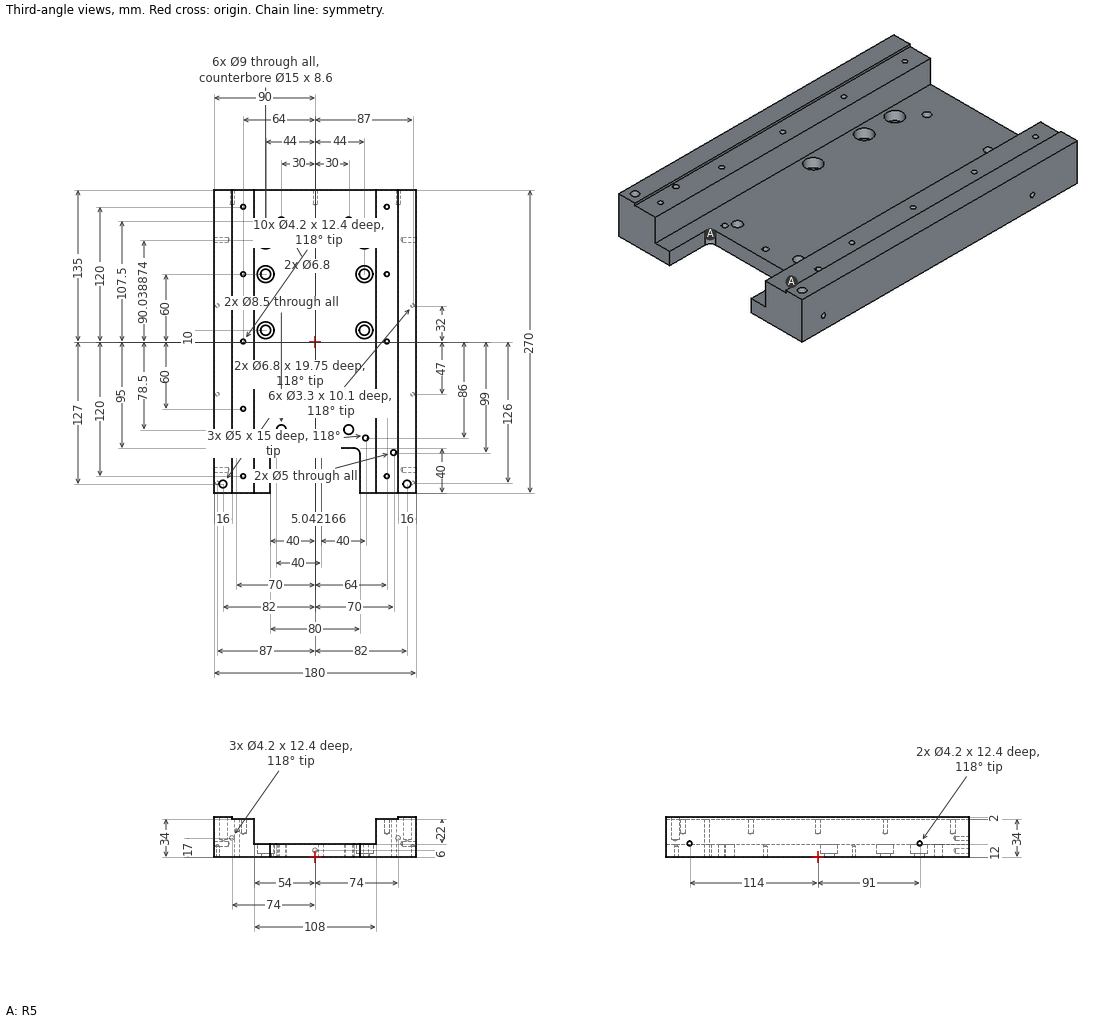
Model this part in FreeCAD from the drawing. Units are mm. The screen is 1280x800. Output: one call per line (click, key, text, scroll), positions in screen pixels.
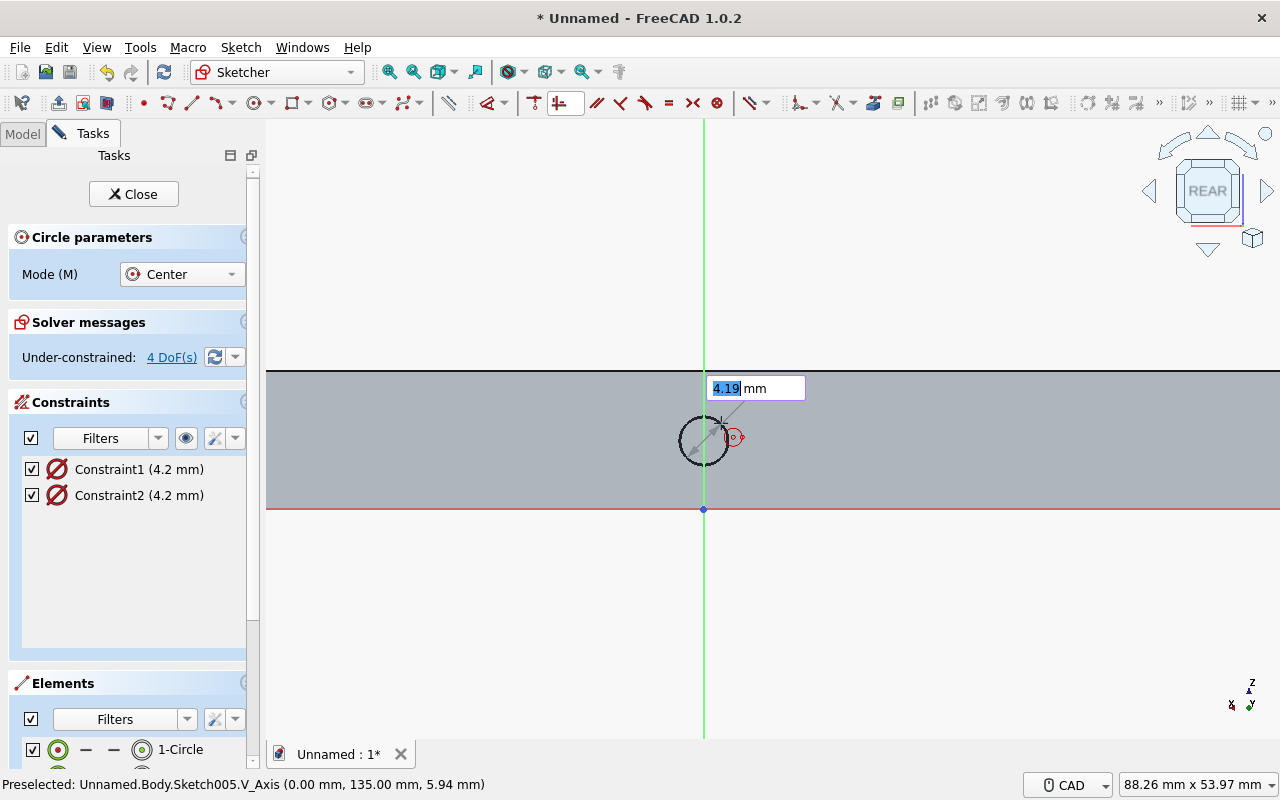
text(4.2)
key(Return)
key(Escape)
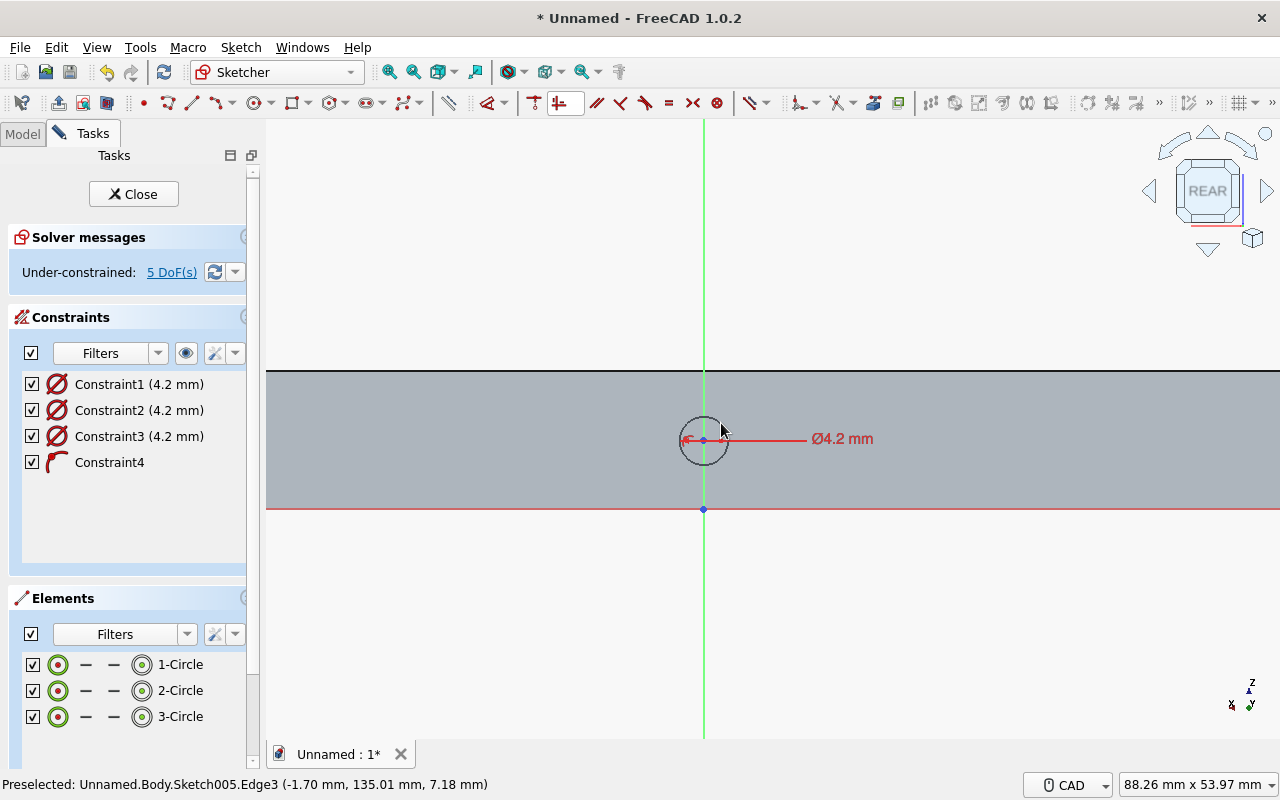
scroll(705, 442, down, 6)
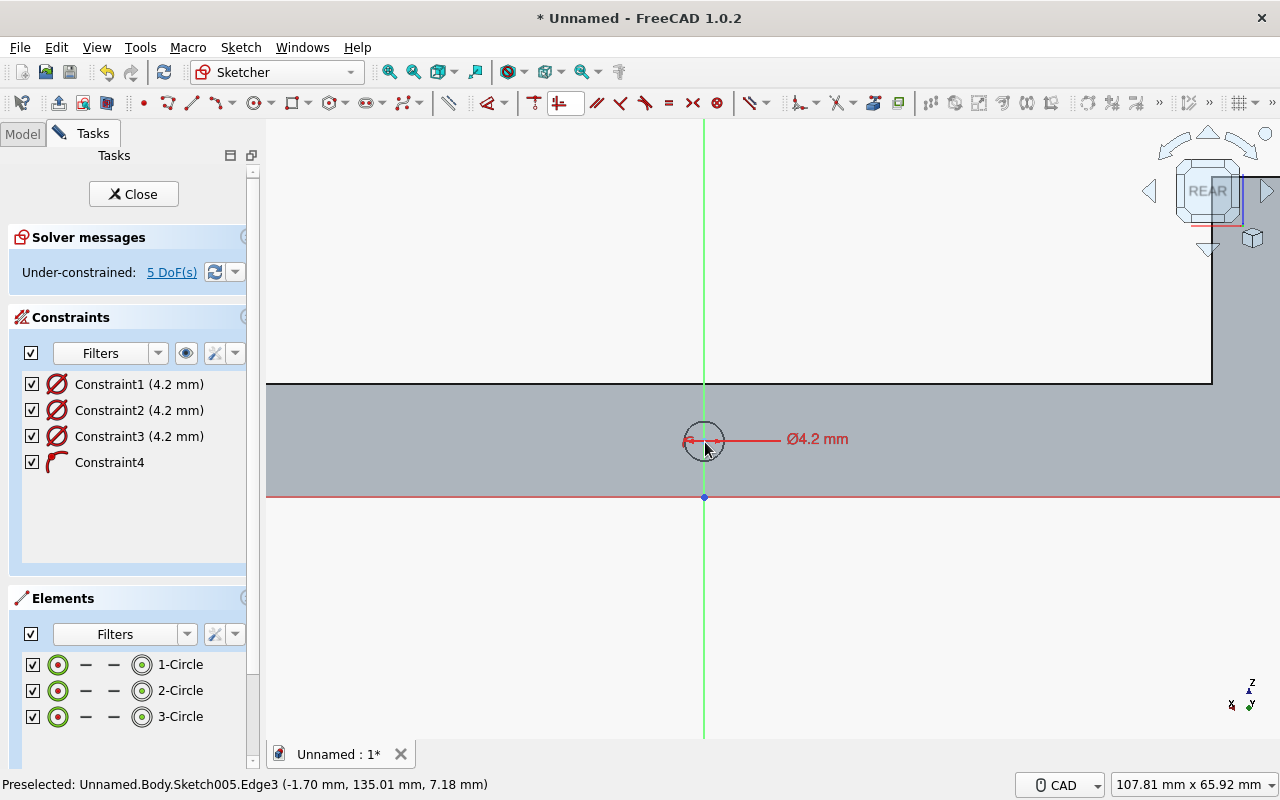
click(961, 404)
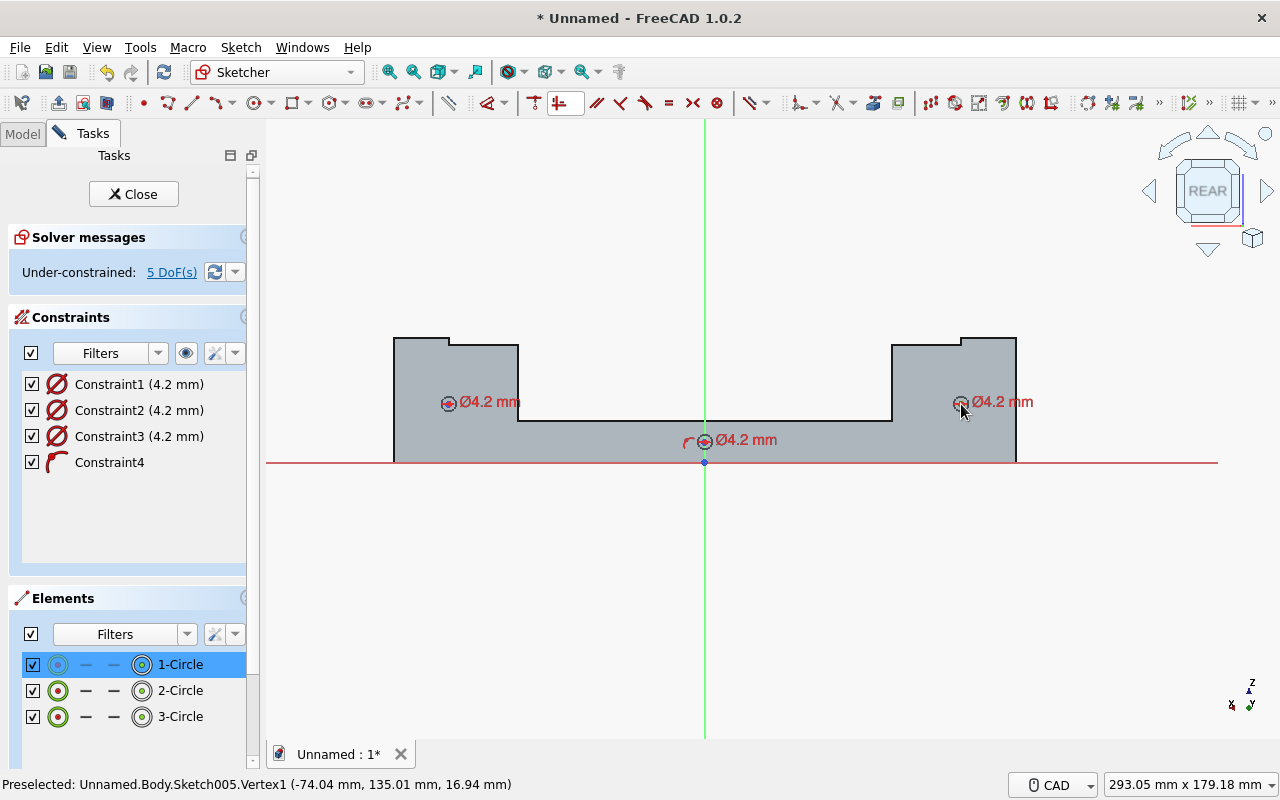
click(449, 404)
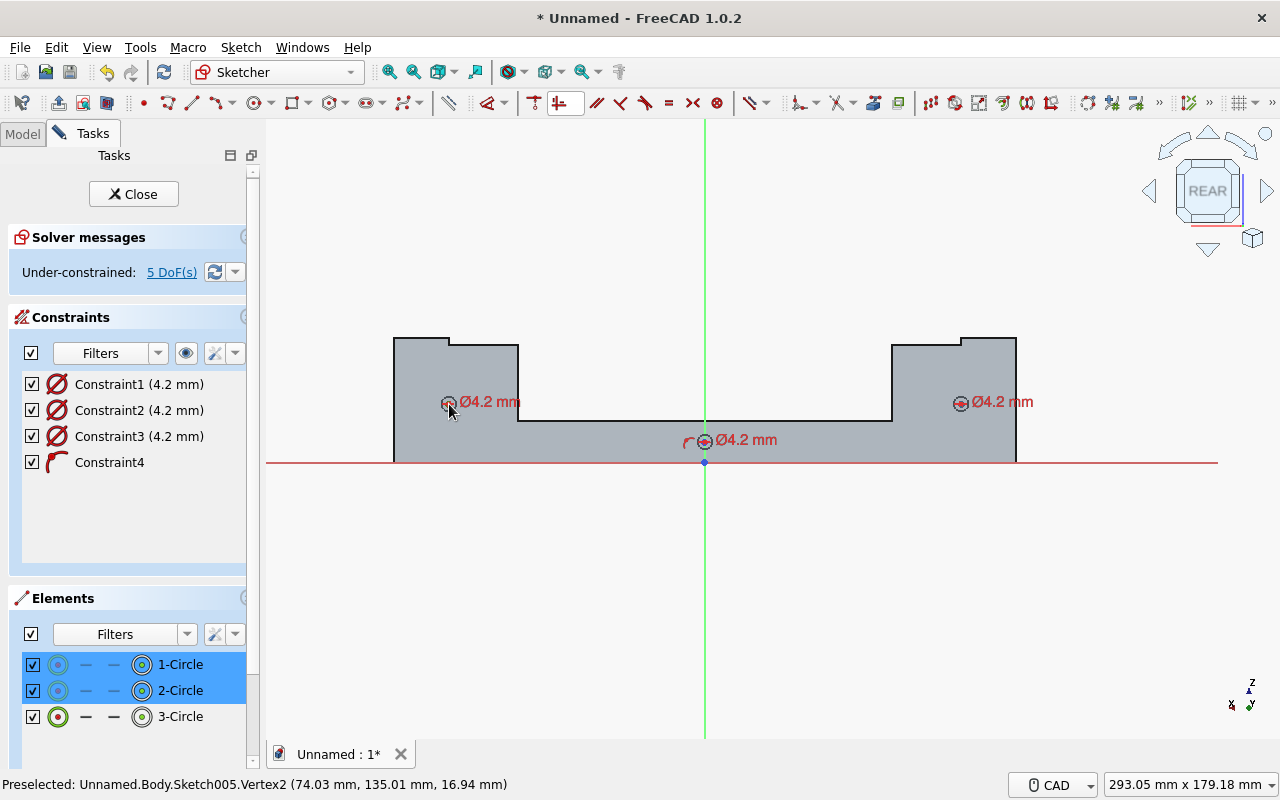
key(h)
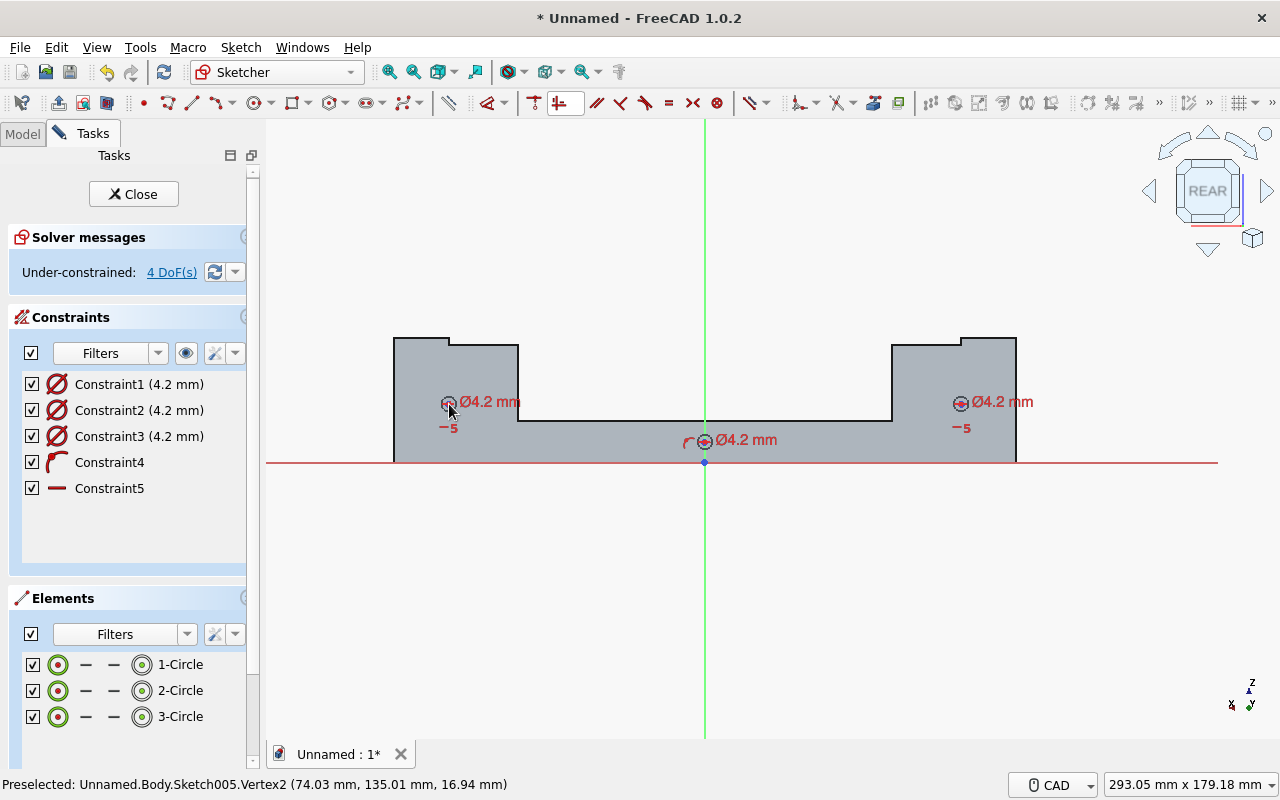
click(488, 104)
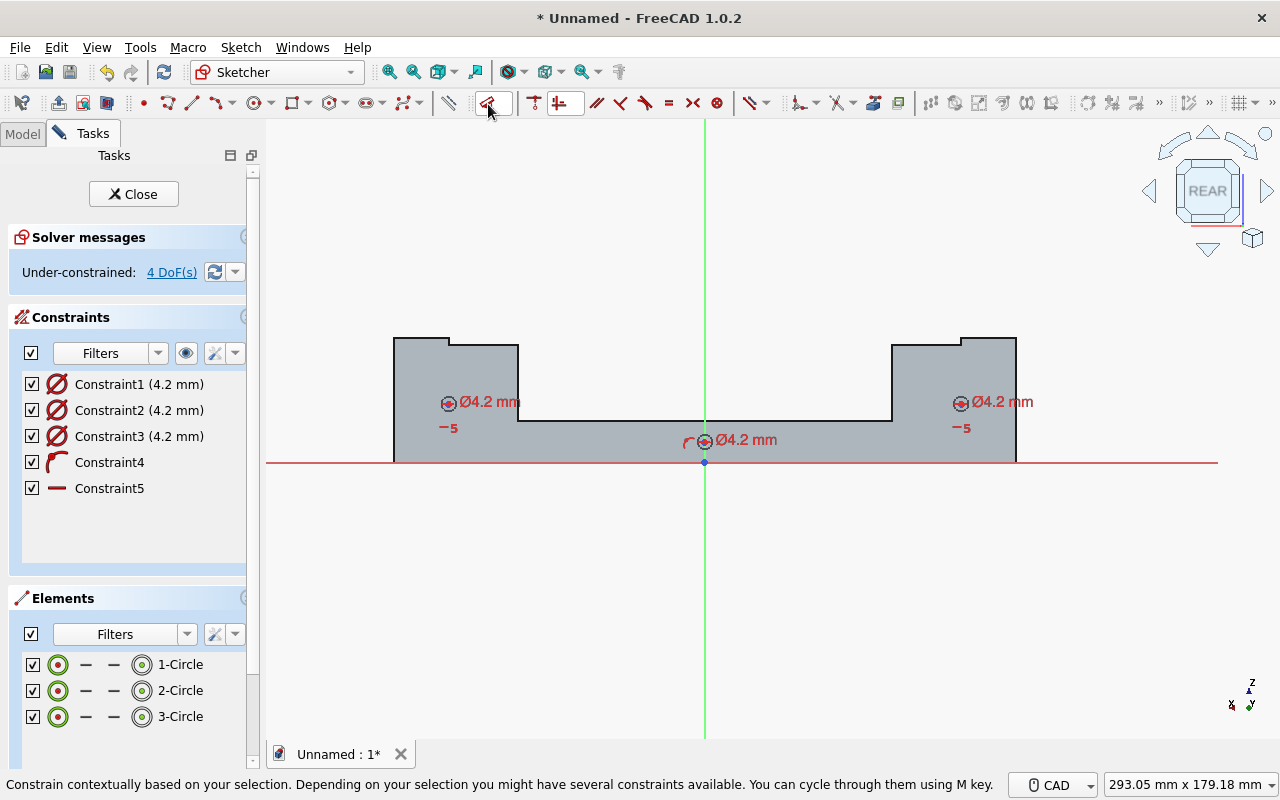
scroll(705, 442, up, 4)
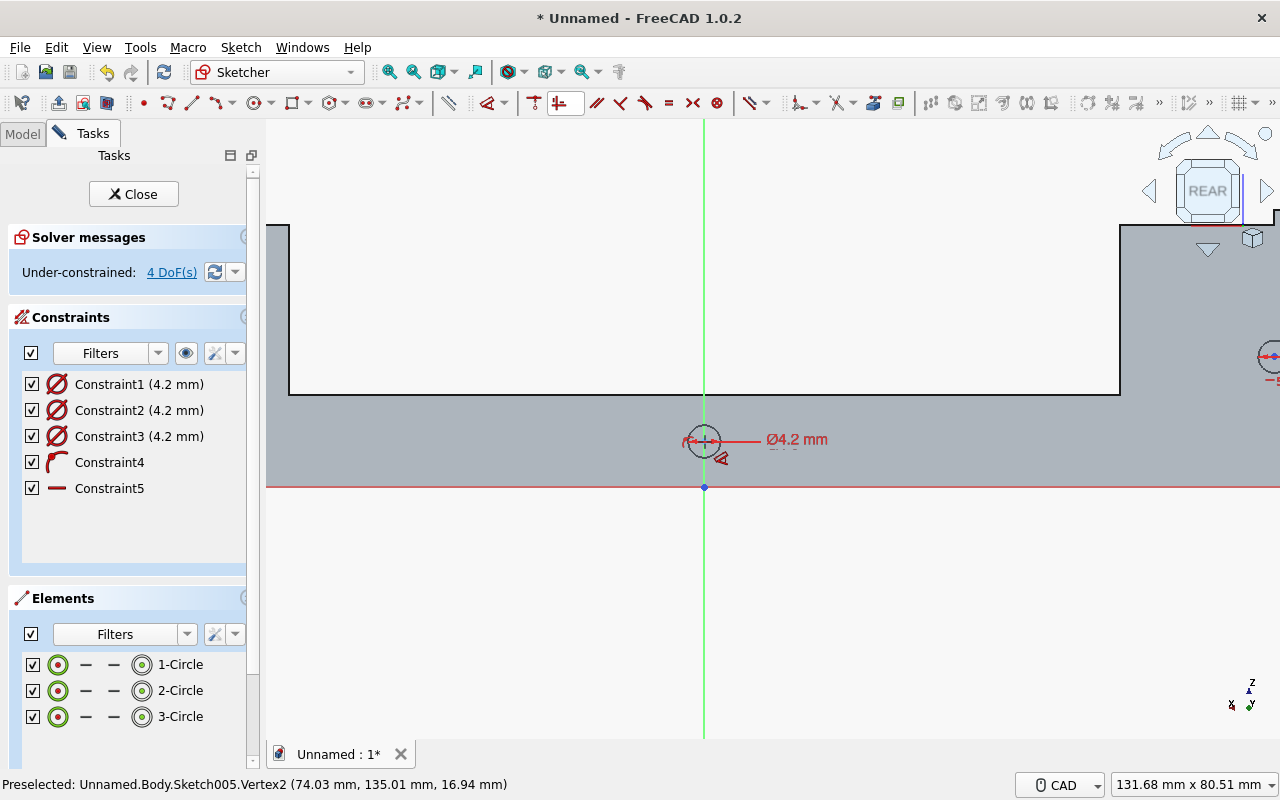
click(704, 442)
click(738, 464)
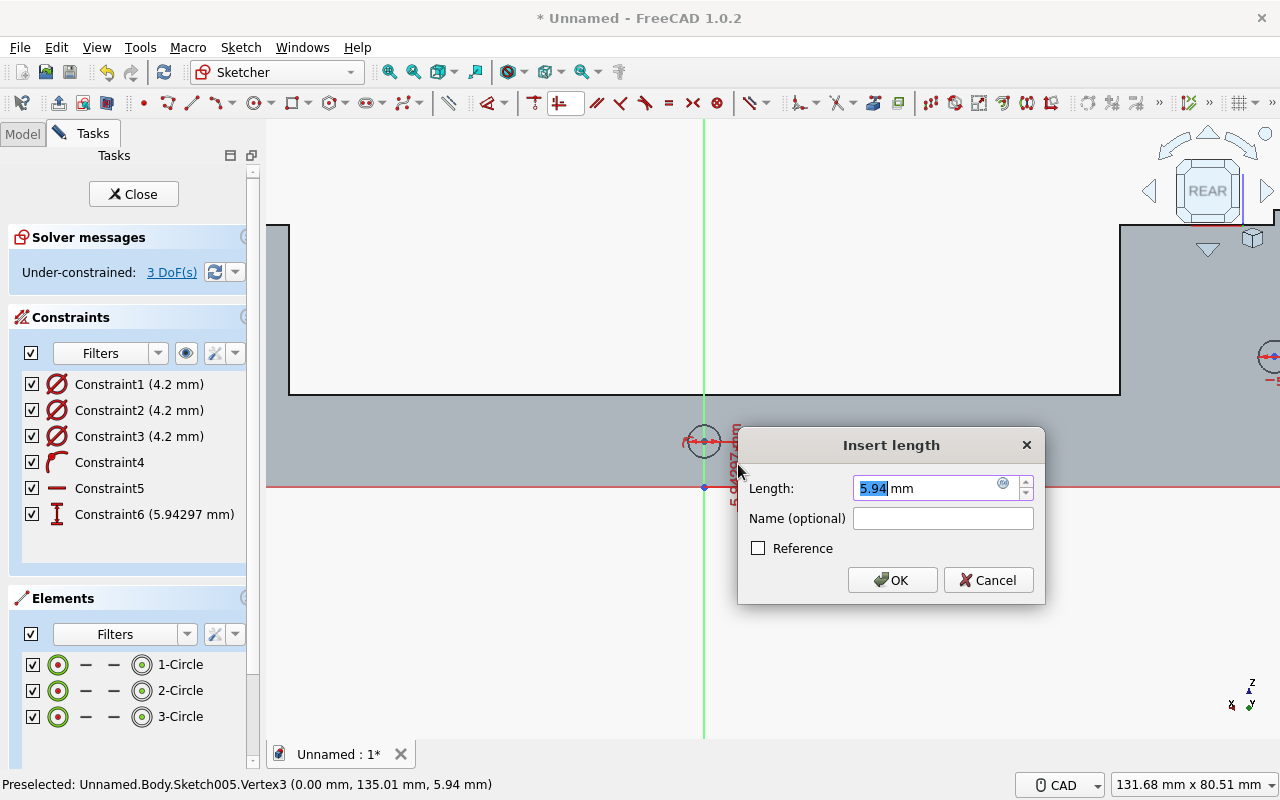
text(6)
key(Return)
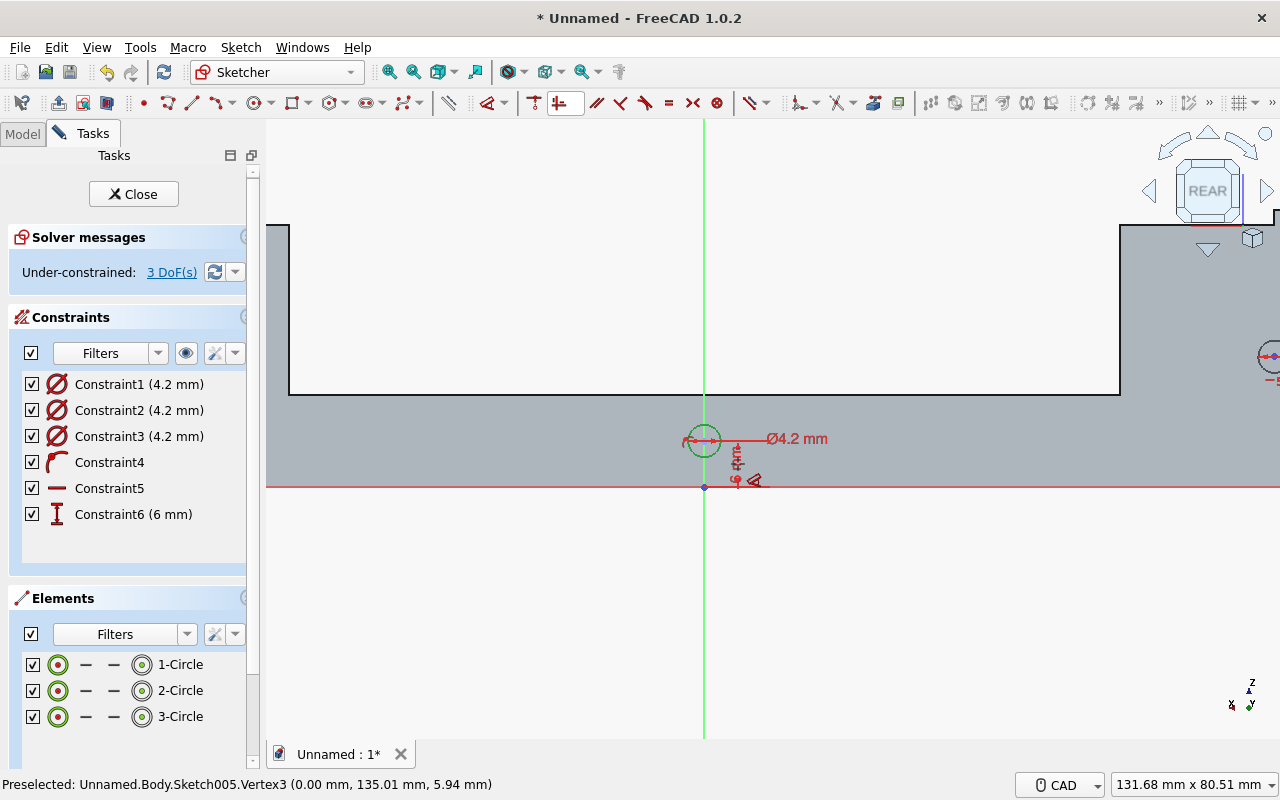
scroll(705, 441, down, 4)